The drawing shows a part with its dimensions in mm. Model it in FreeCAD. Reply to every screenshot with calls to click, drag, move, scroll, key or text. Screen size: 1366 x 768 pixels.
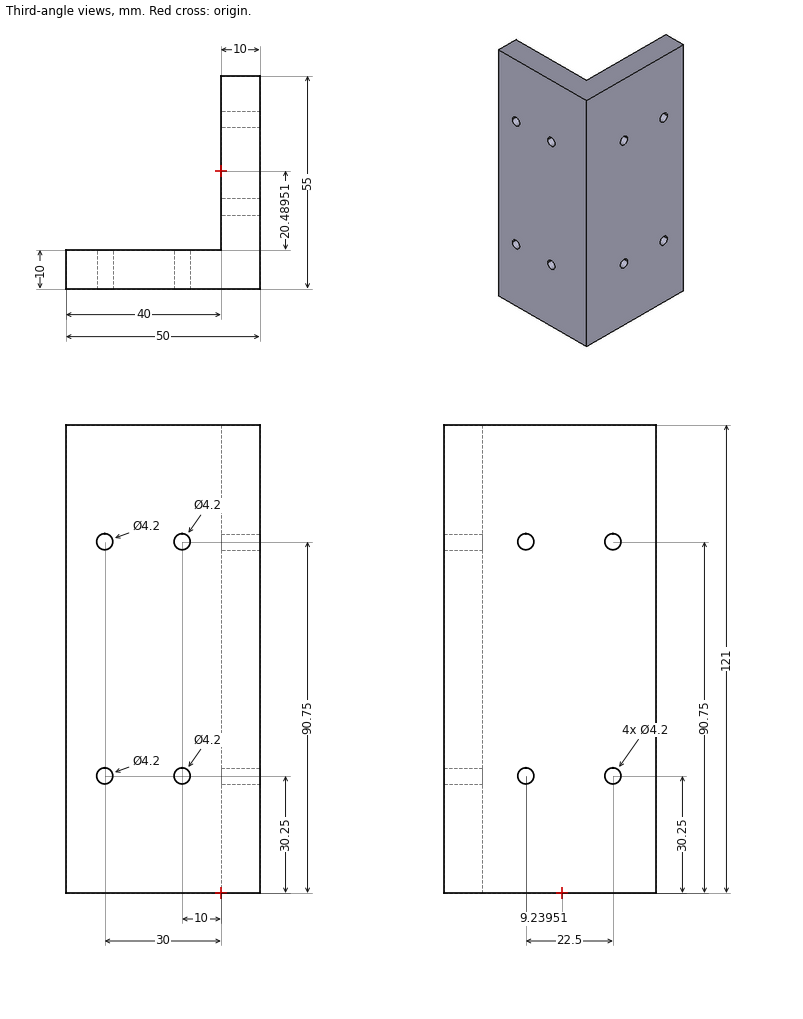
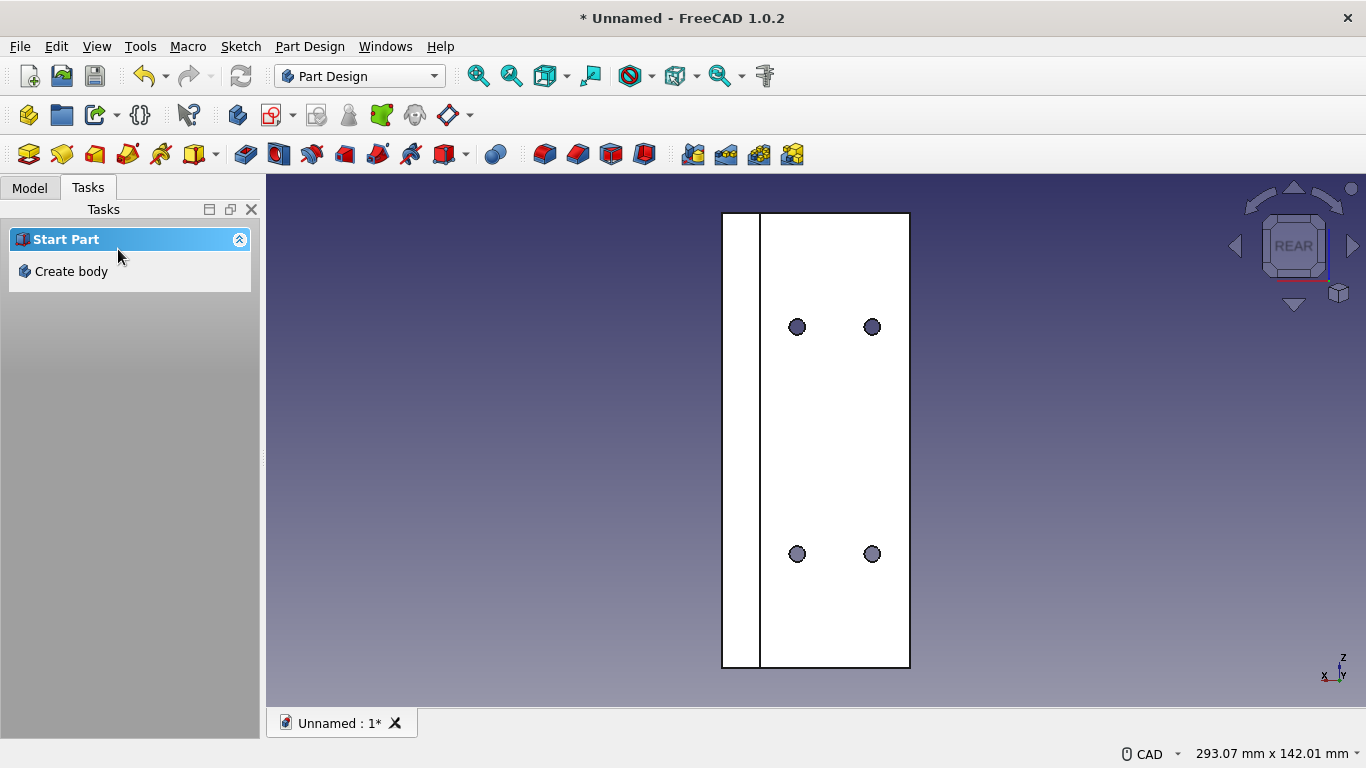
click(270, 116)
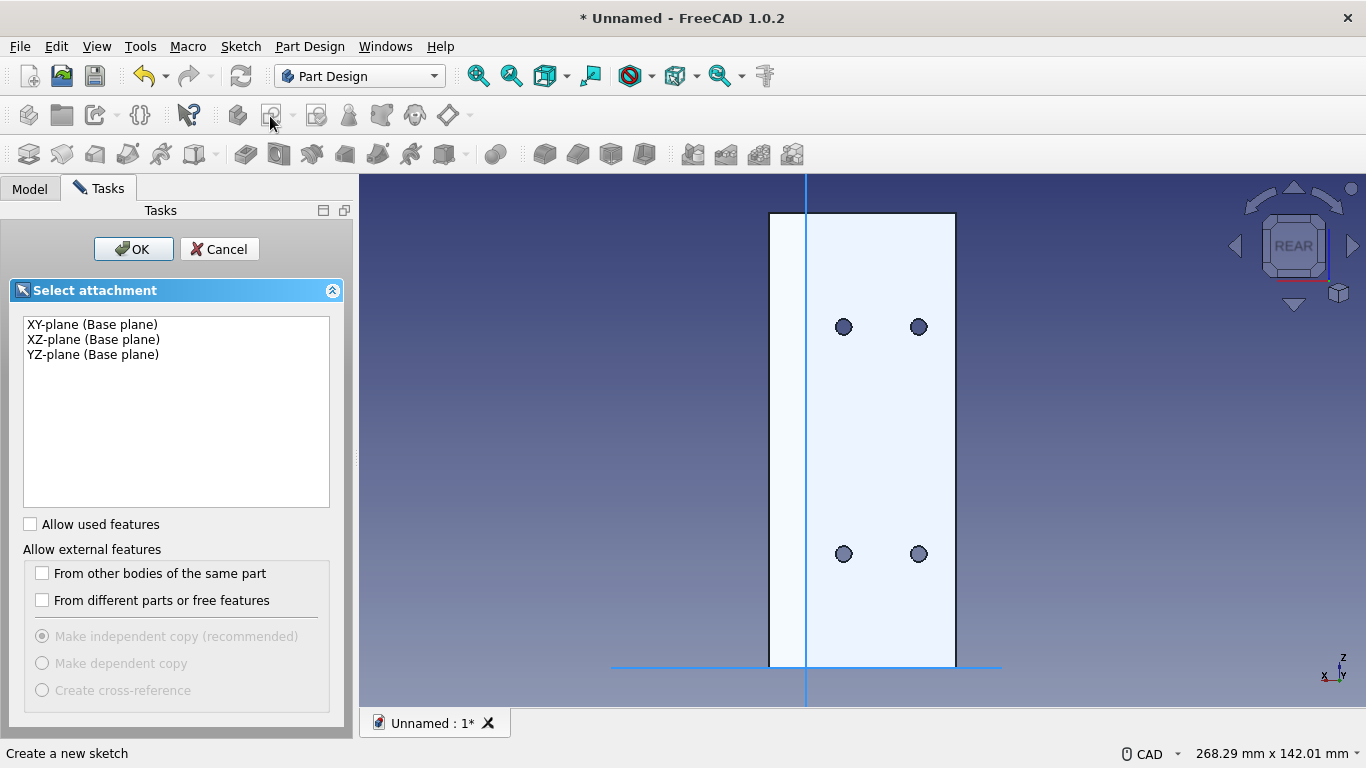
click(84, 354)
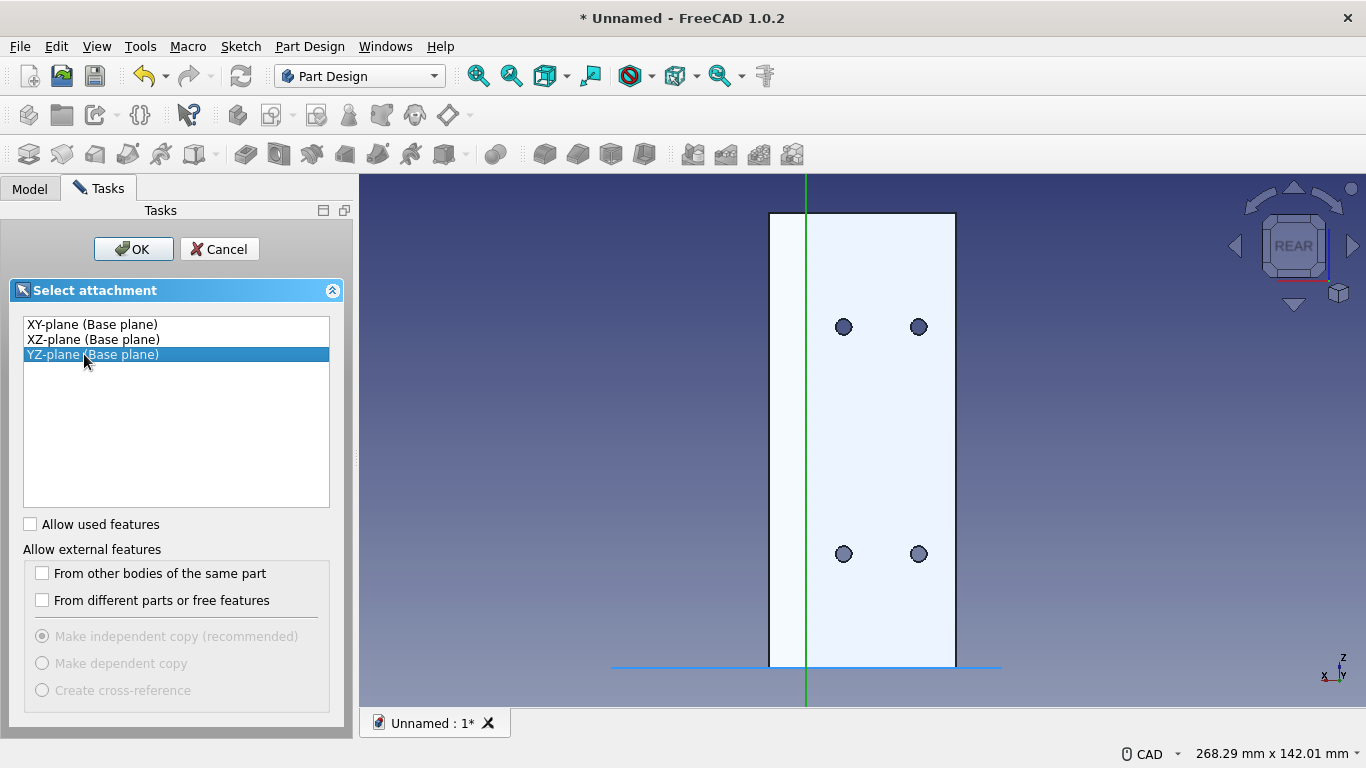
click(134, 249)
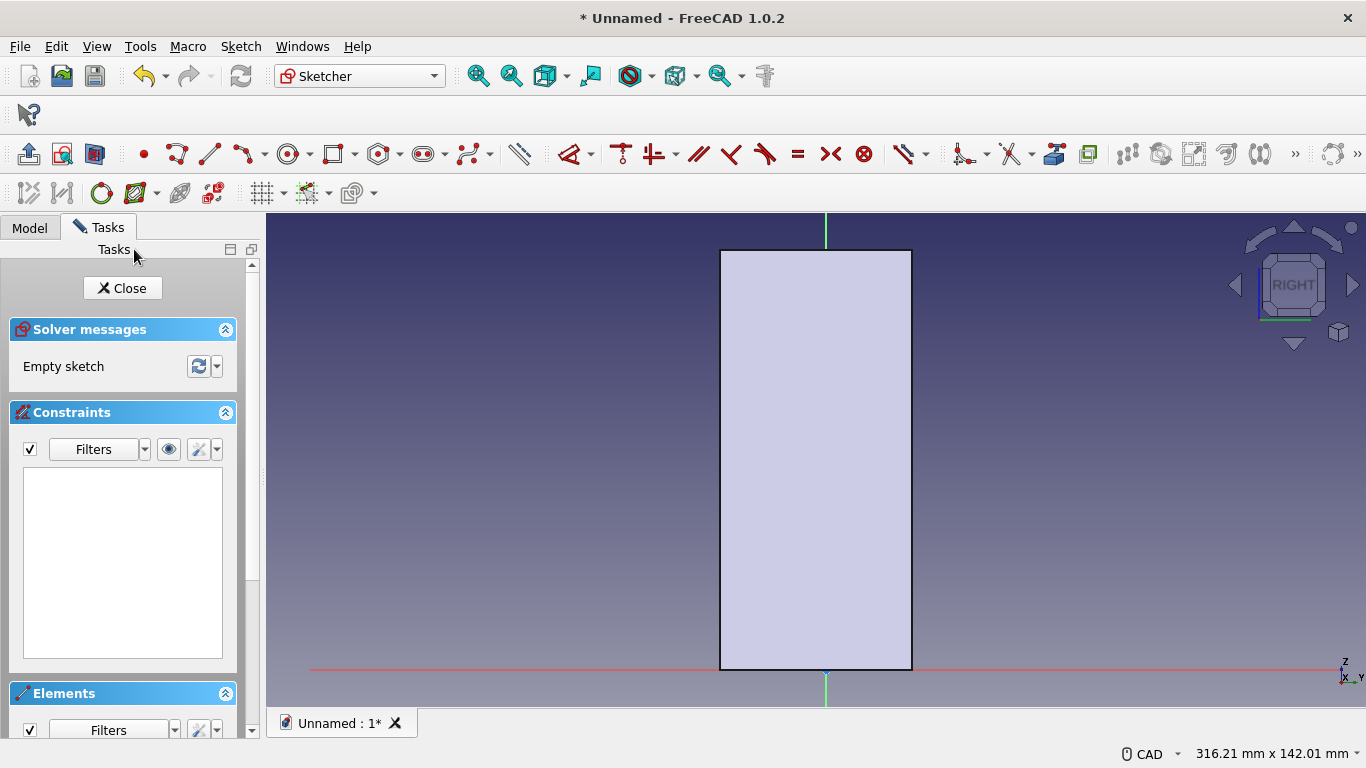
click(95, 154)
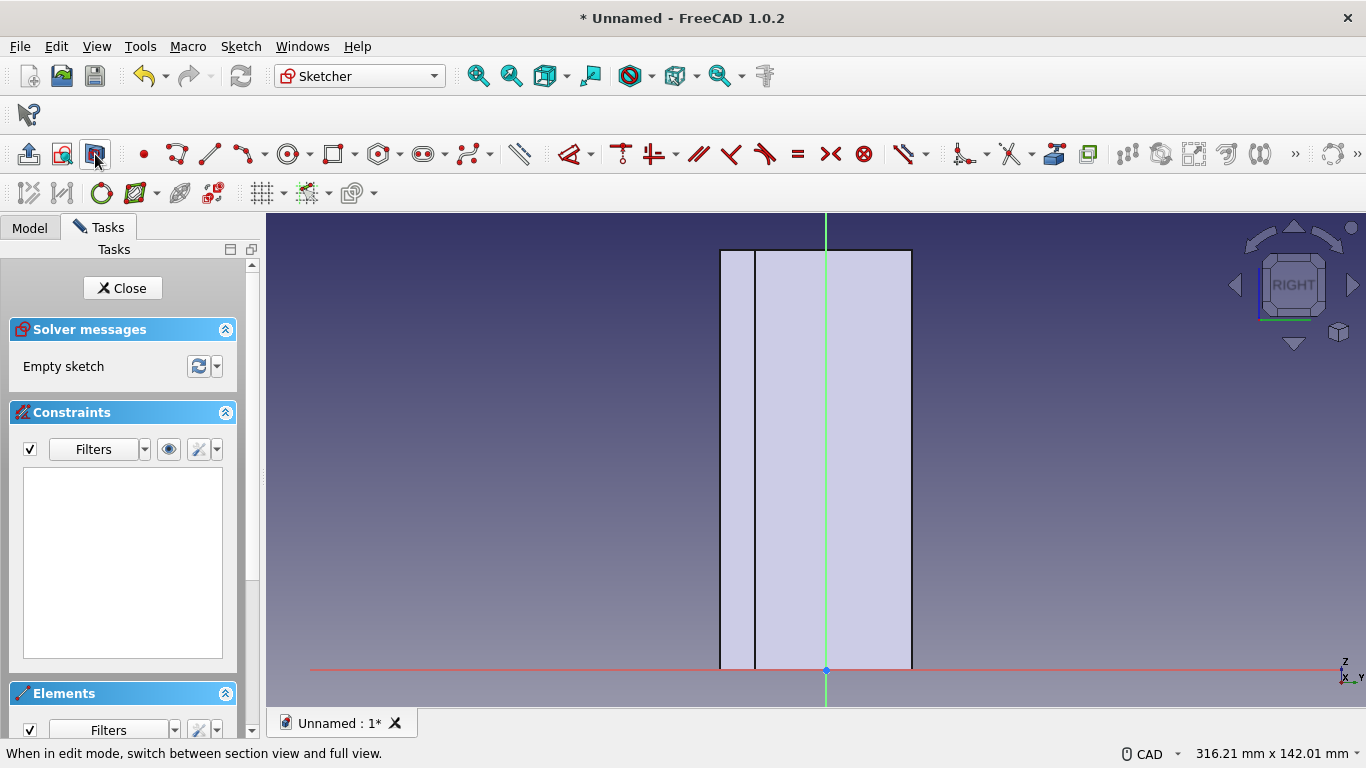
scroll(360, 241, down, 1)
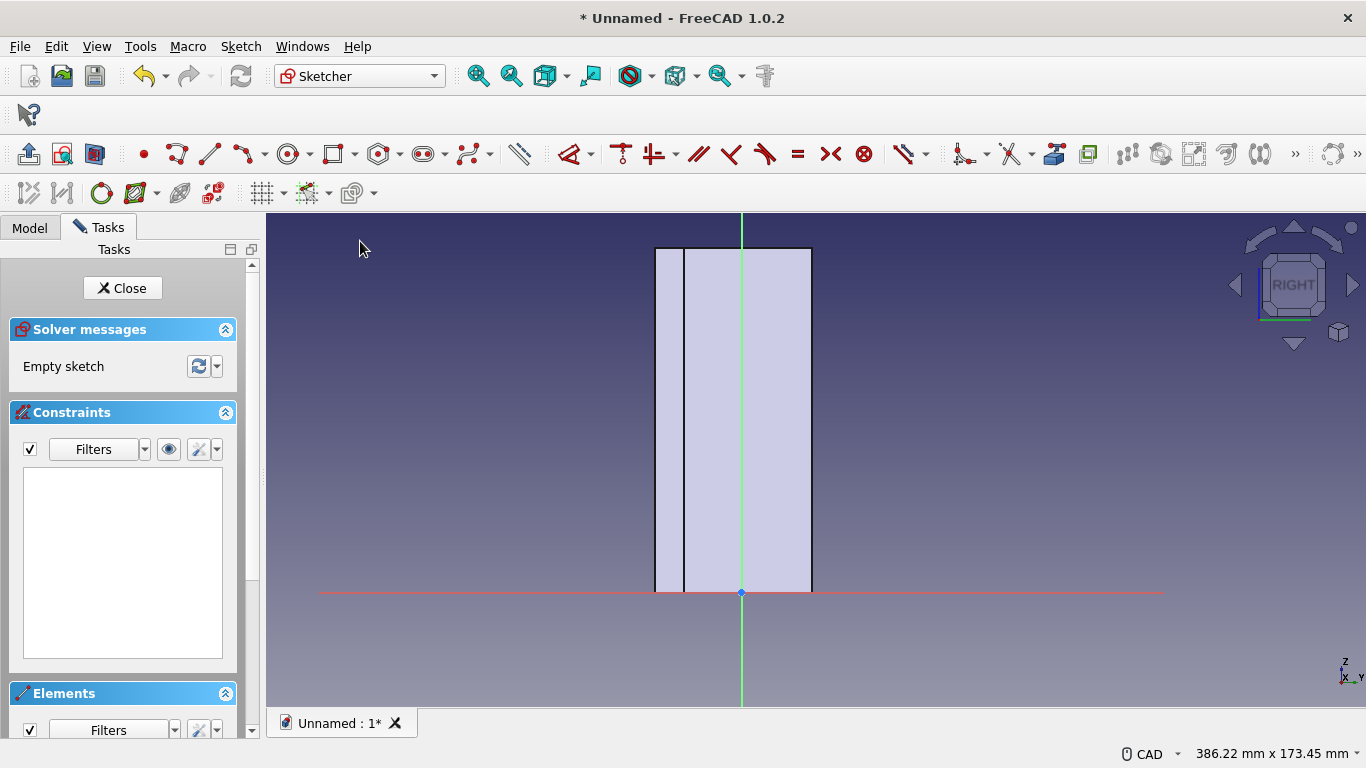
click(288, 154)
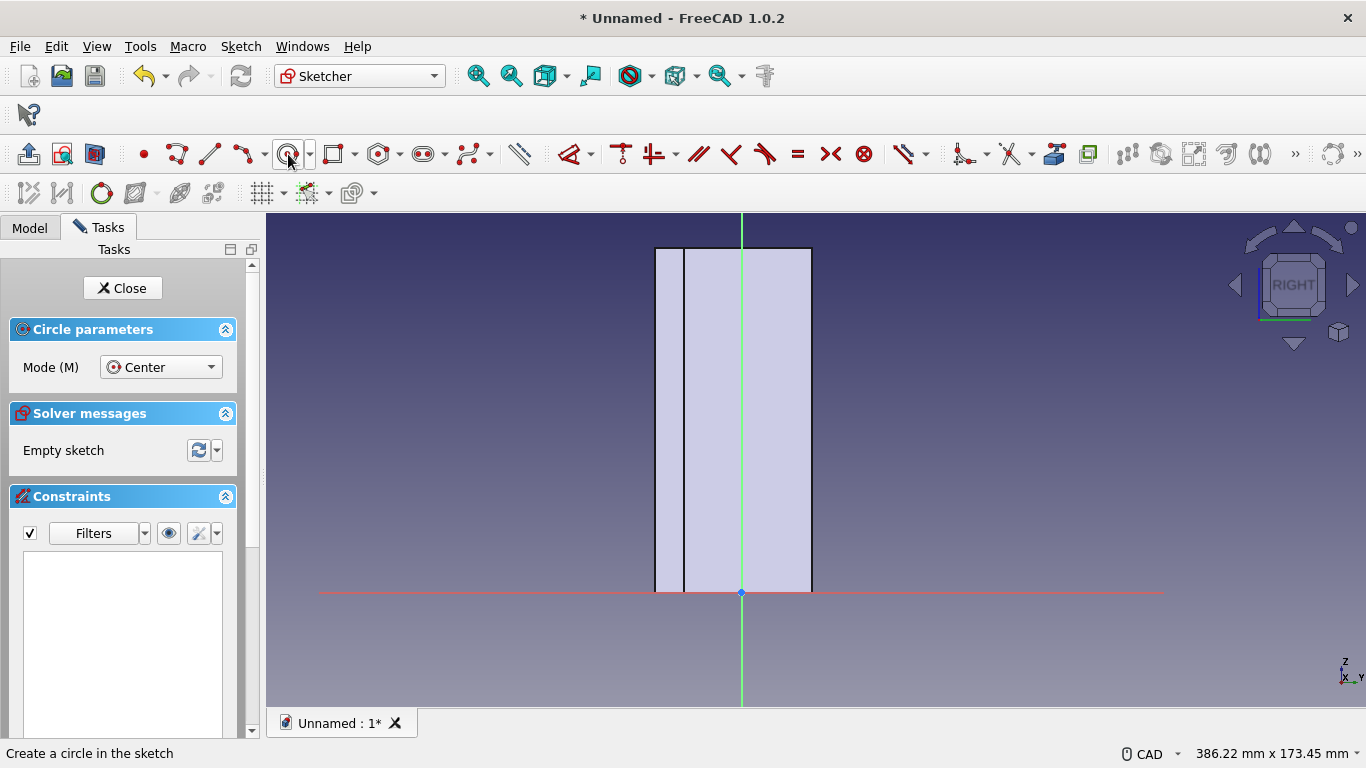
scroll(780, 506, up, 7)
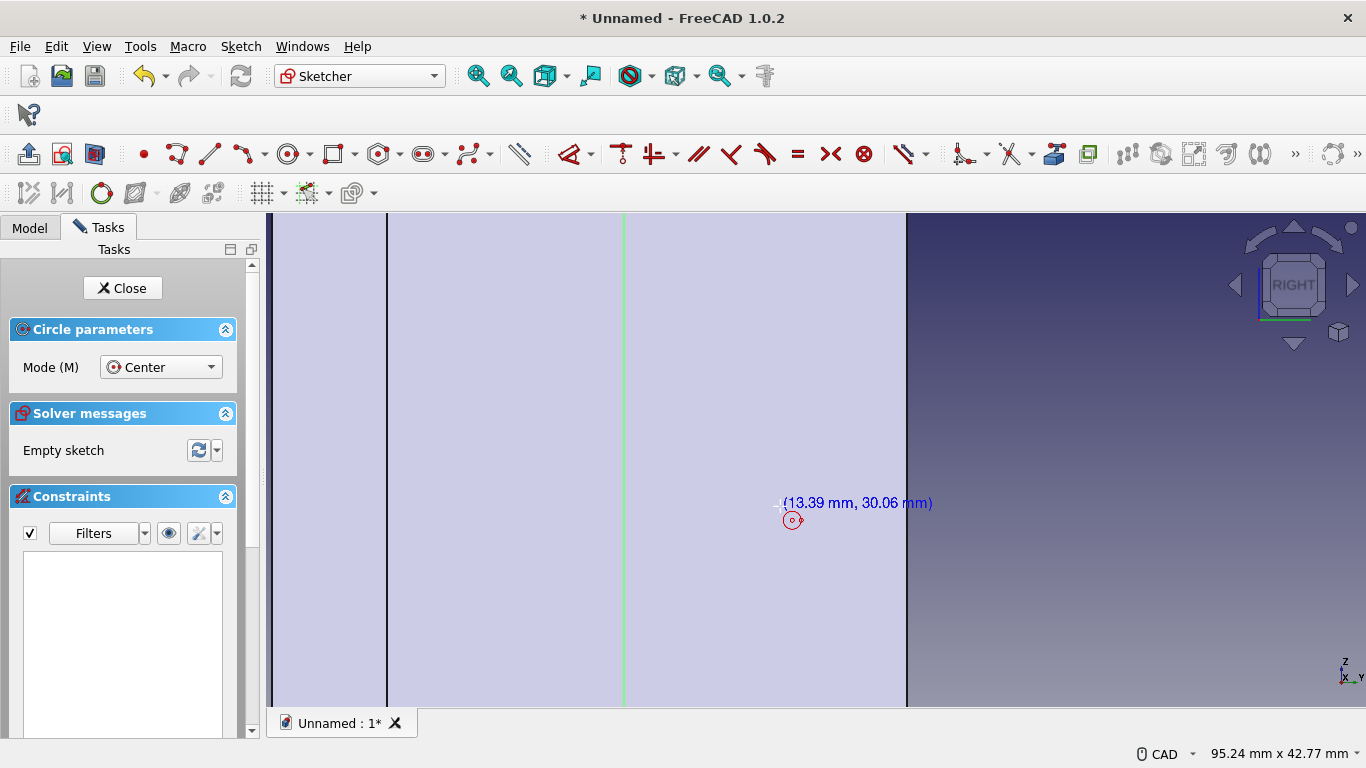
scroll(791, 521, down, 6)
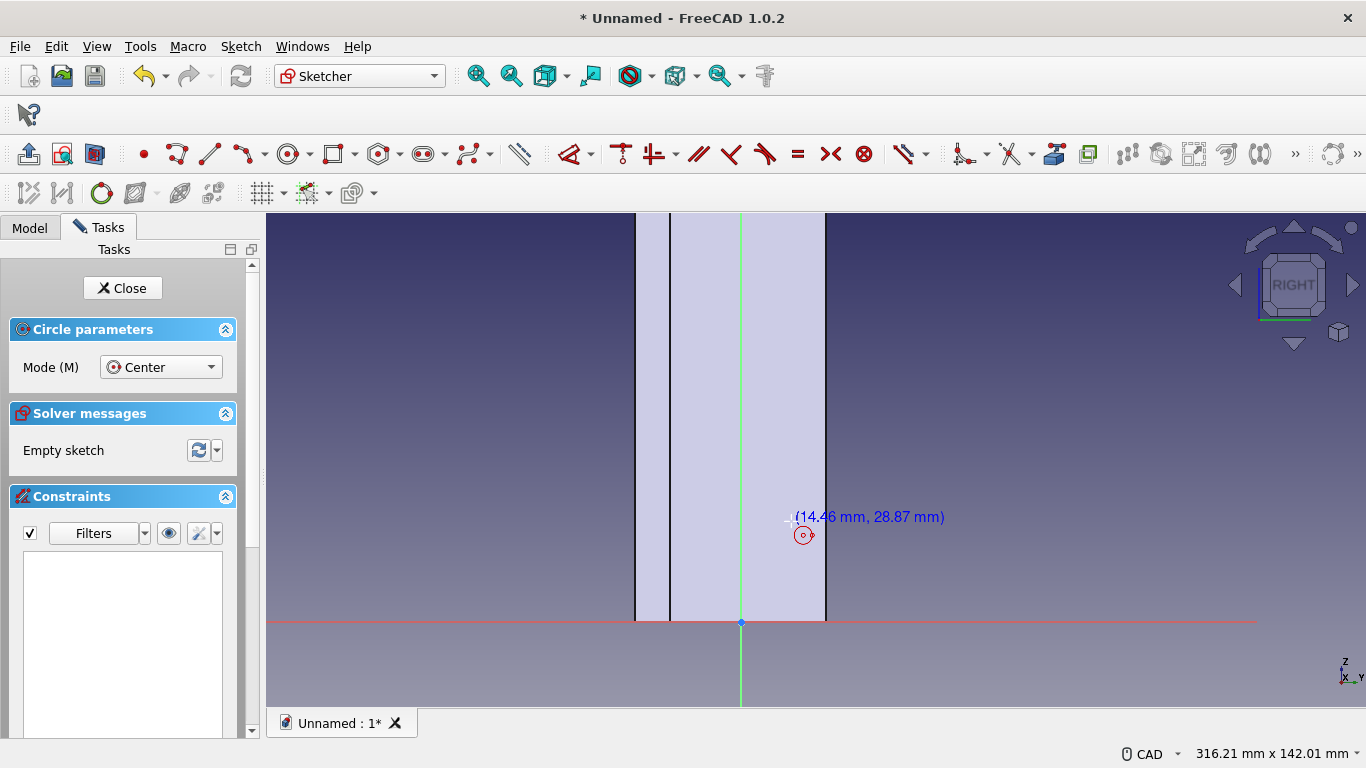
click(787, 517)
move(792, 512)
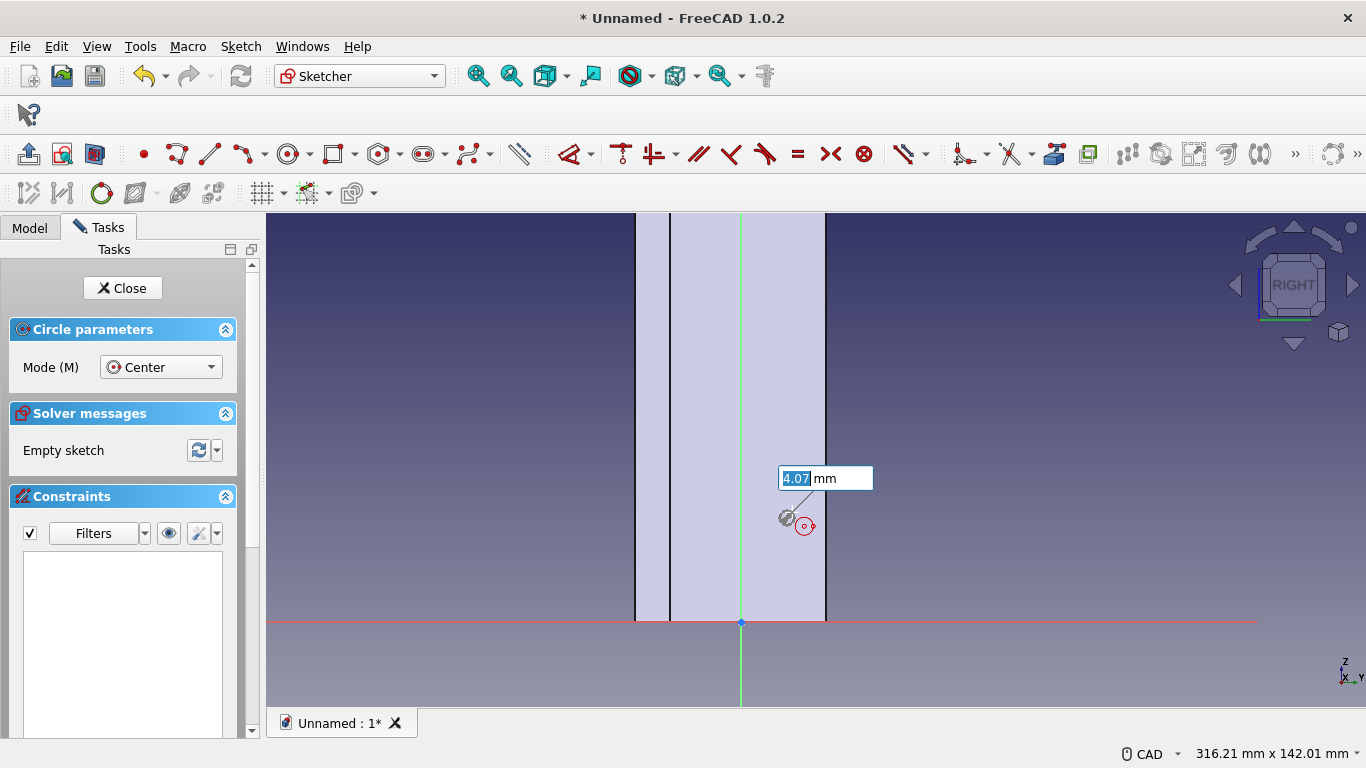
text(4.2)
key(Return)